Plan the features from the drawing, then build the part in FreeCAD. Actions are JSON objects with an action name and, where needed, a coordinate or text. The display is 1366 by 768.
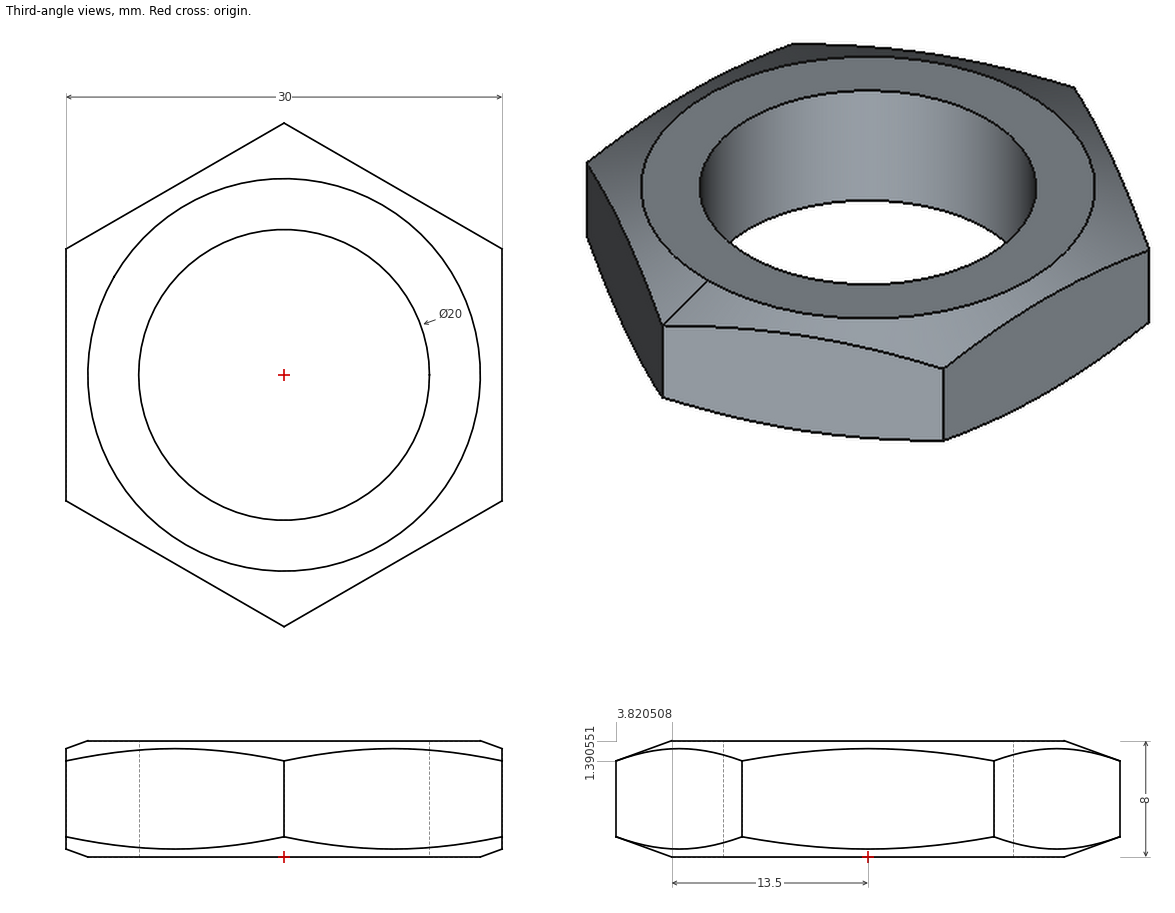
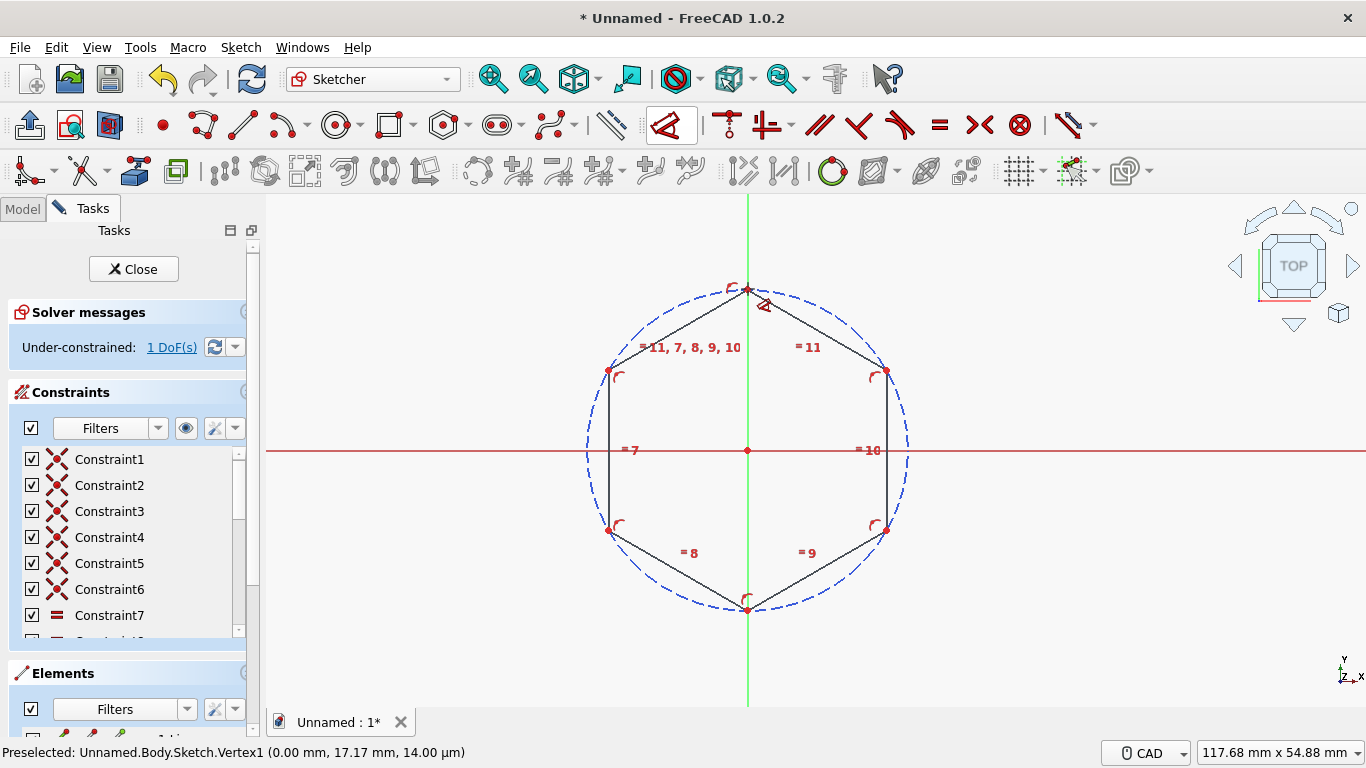
{"action": "left_click", "coordinate": [609, 370]}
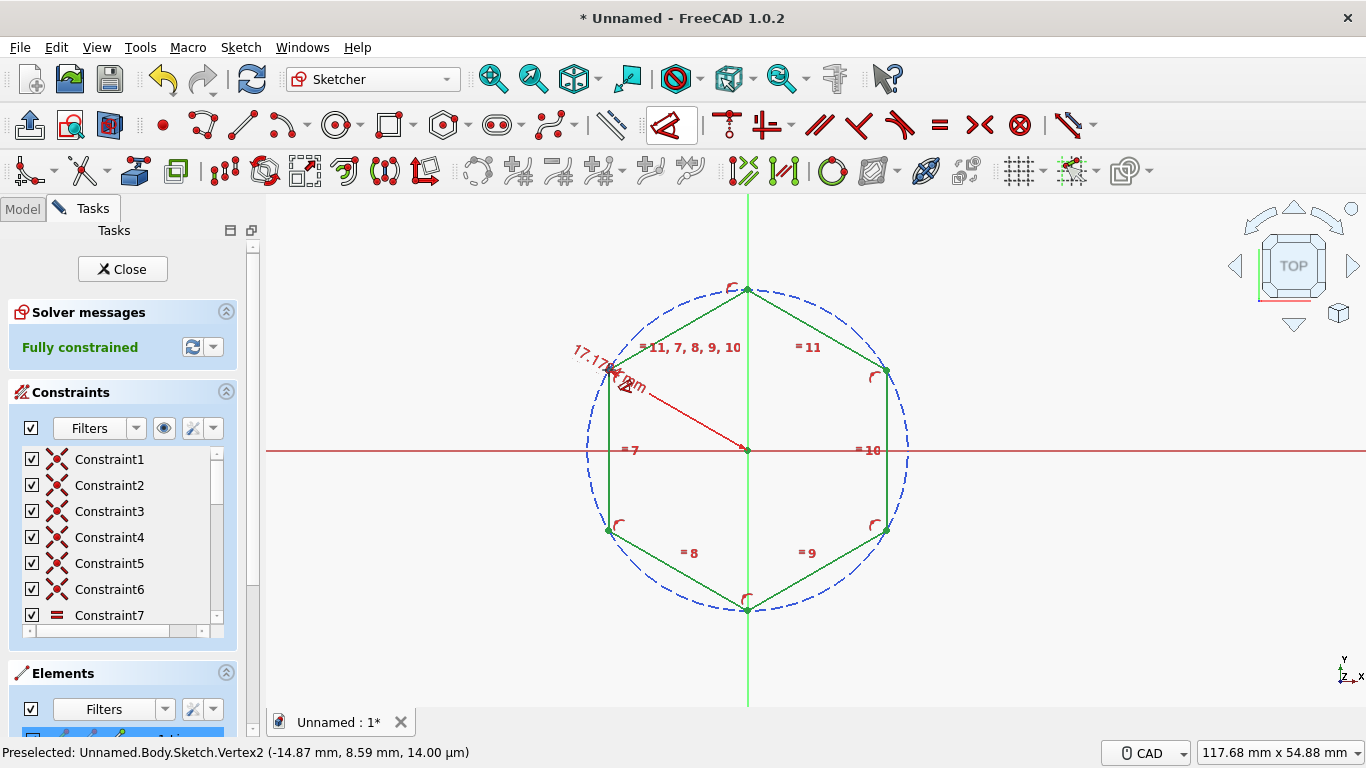
{"action": "left_click", "coordinate": [887, 531]}
{"action": "left_click", "coordinate": [684, 613]}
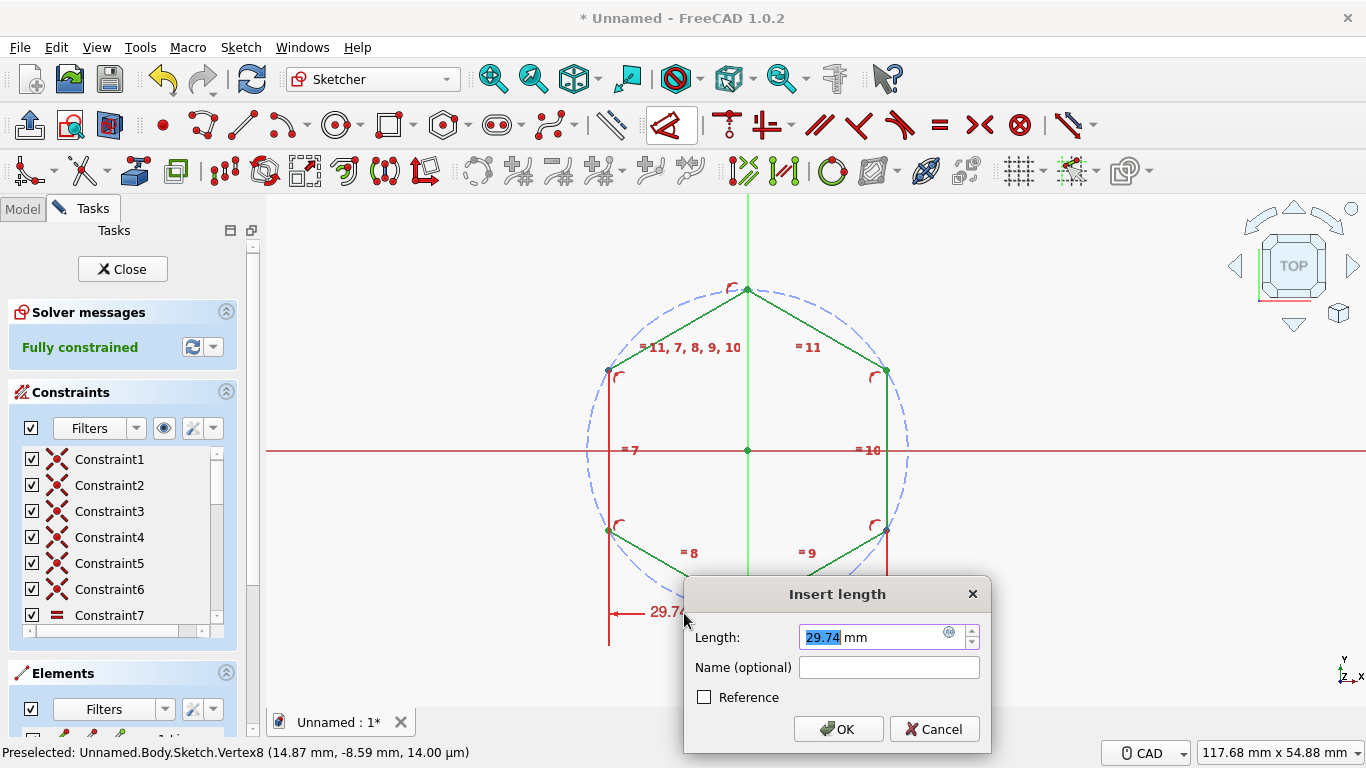
{"action": "type", "text": "30"}
{"action": "key", "text": "Return"}
{"action": "key", "text": "Escape"}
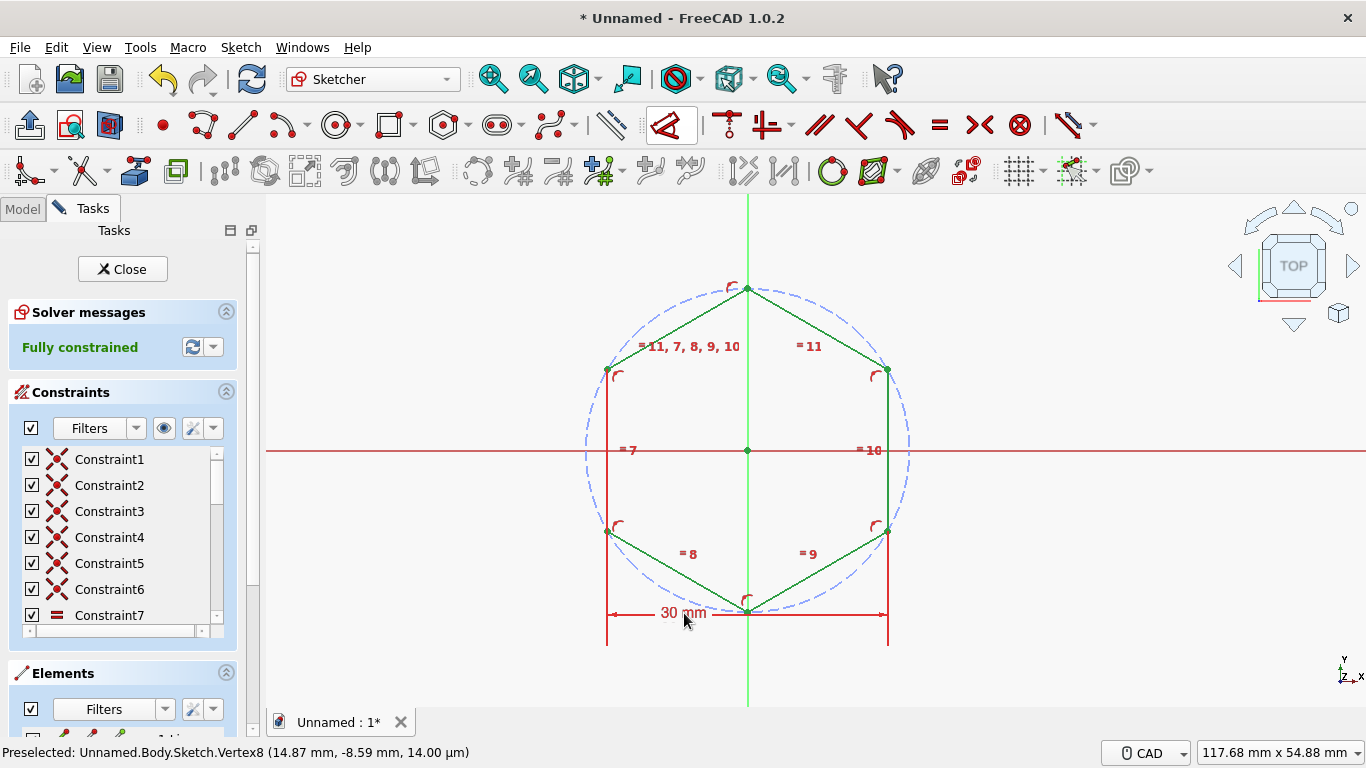
{"action": "left_click", "coordinate": [123, 269]}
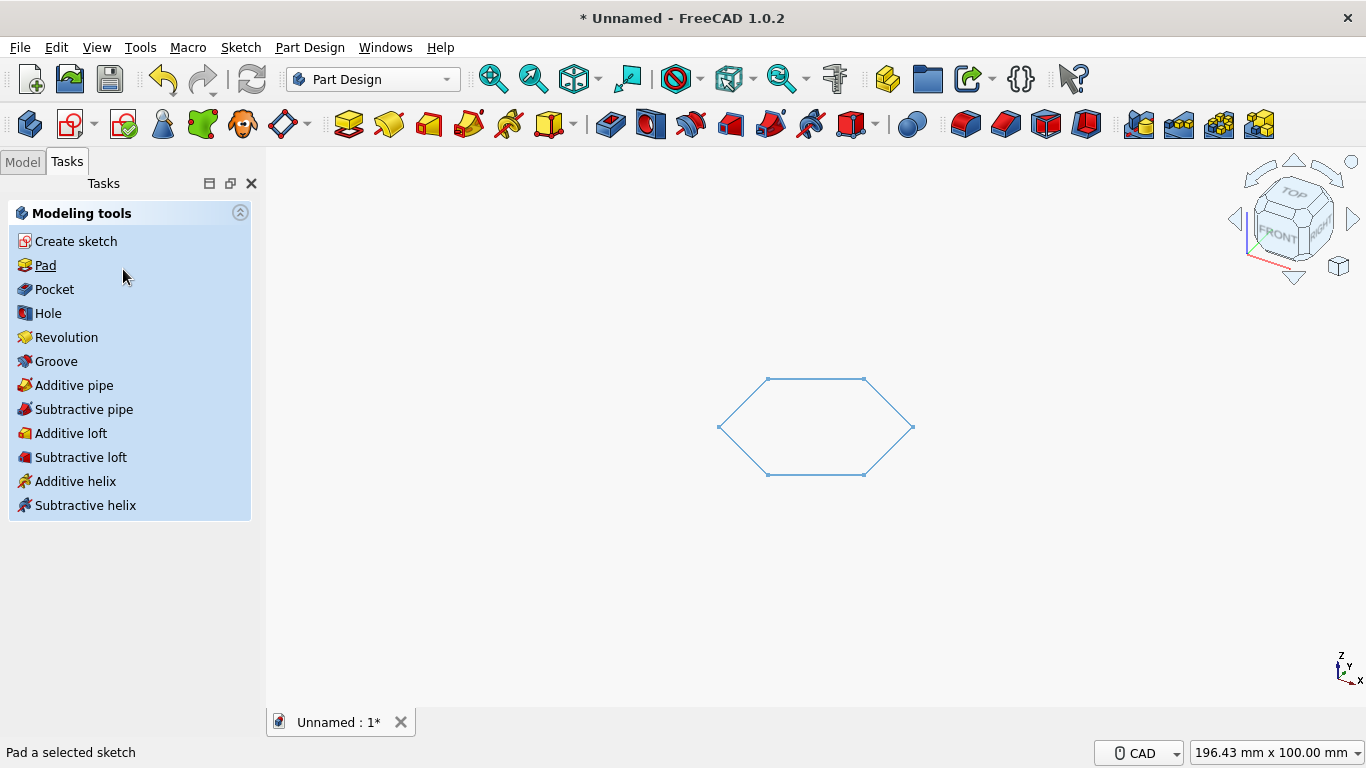
{"action": "left_click", "coordinate": [350, 124]}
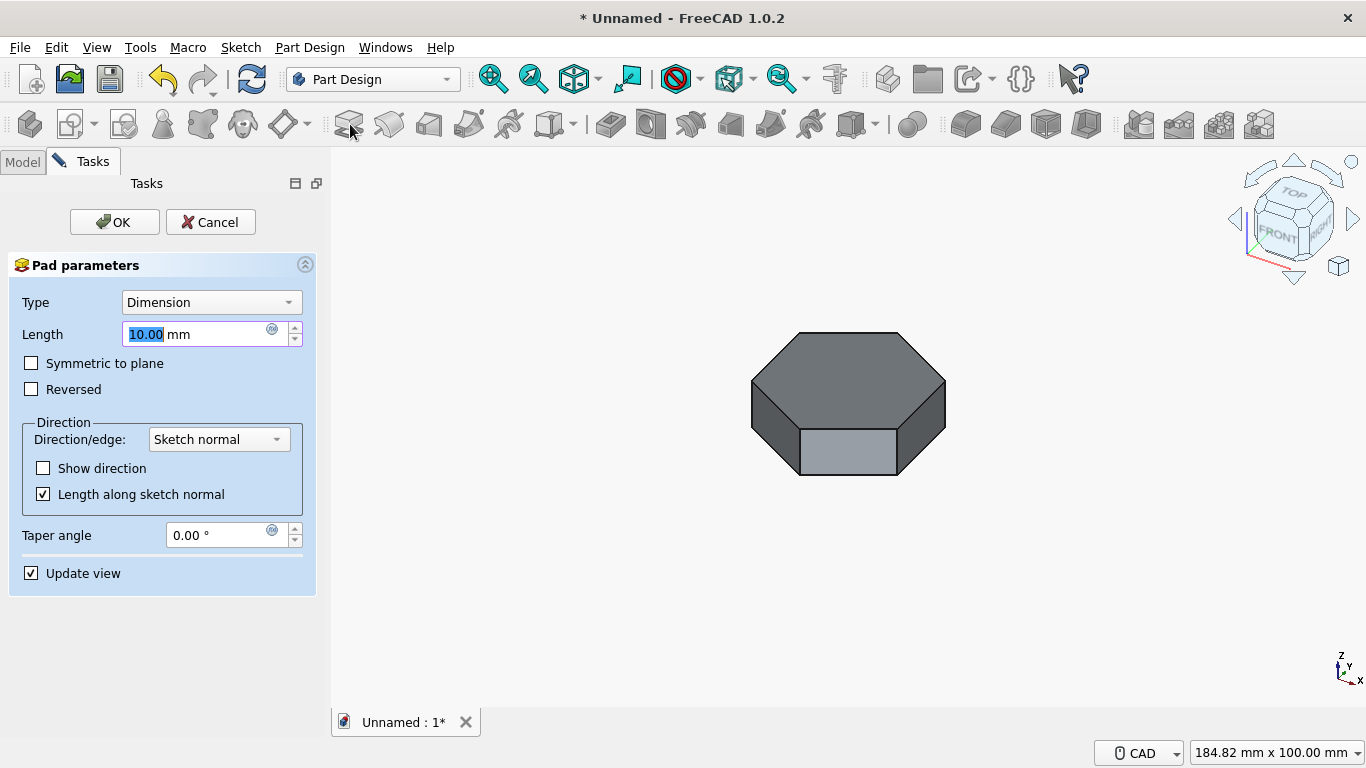
{"action": "type", "text": "8"}
{"action": "key", "text": "Tab"}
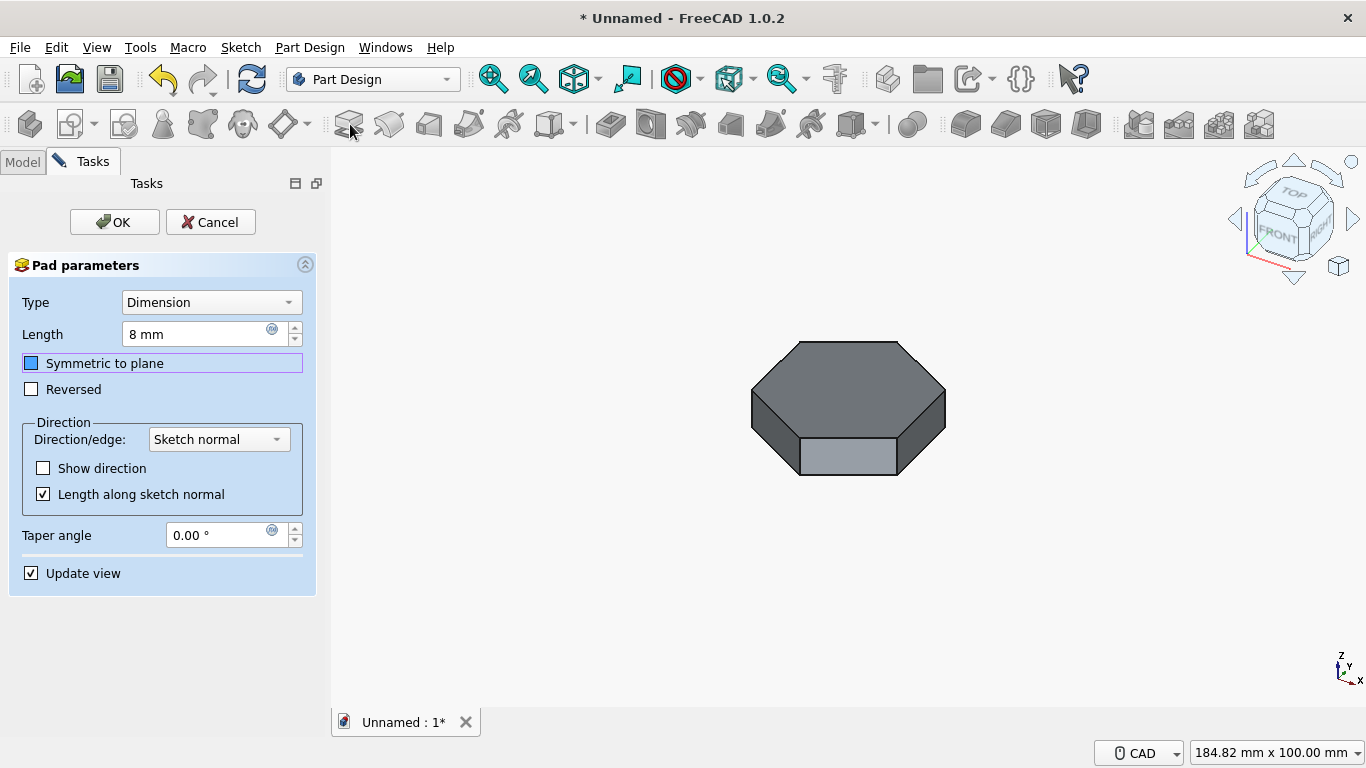
{"action": "left_click", "coordinate": [115, 222]}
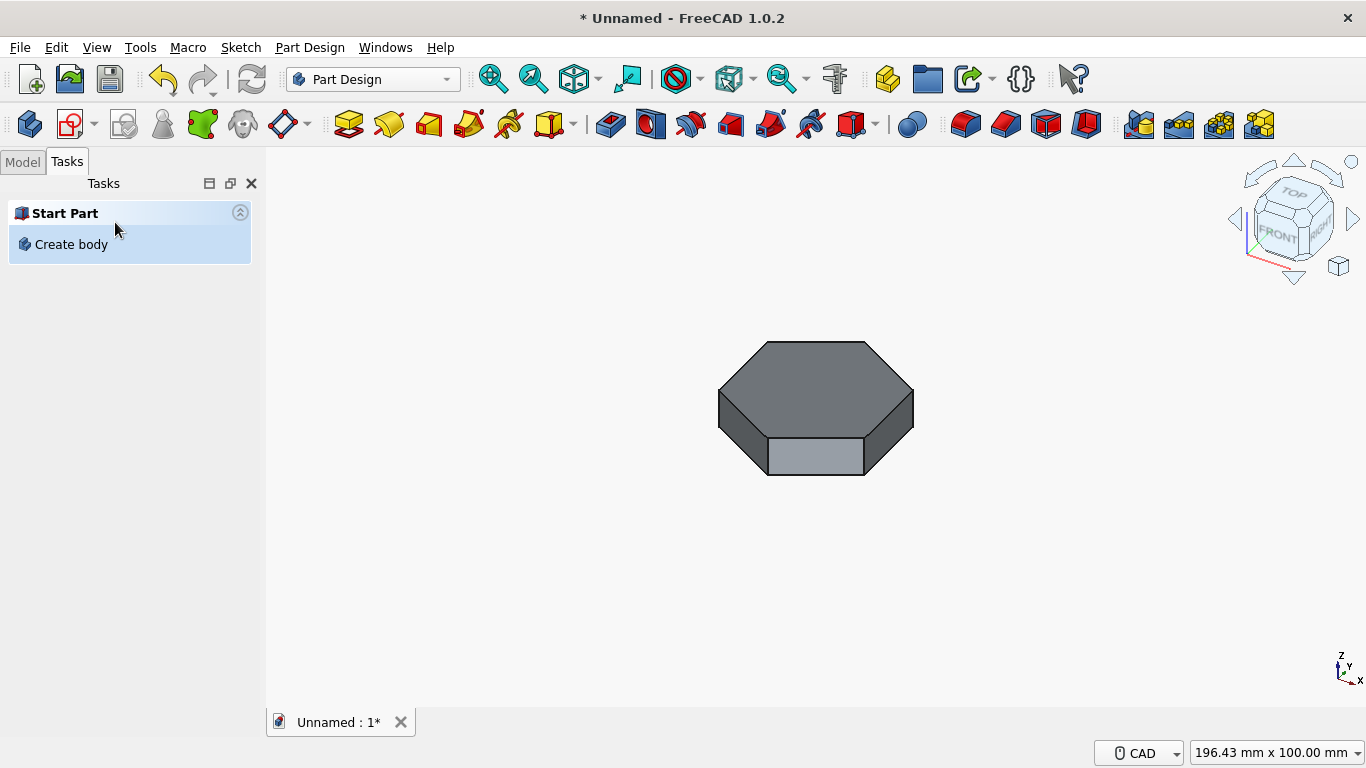
{"action": "left_click", "coordinate": [494, 80]}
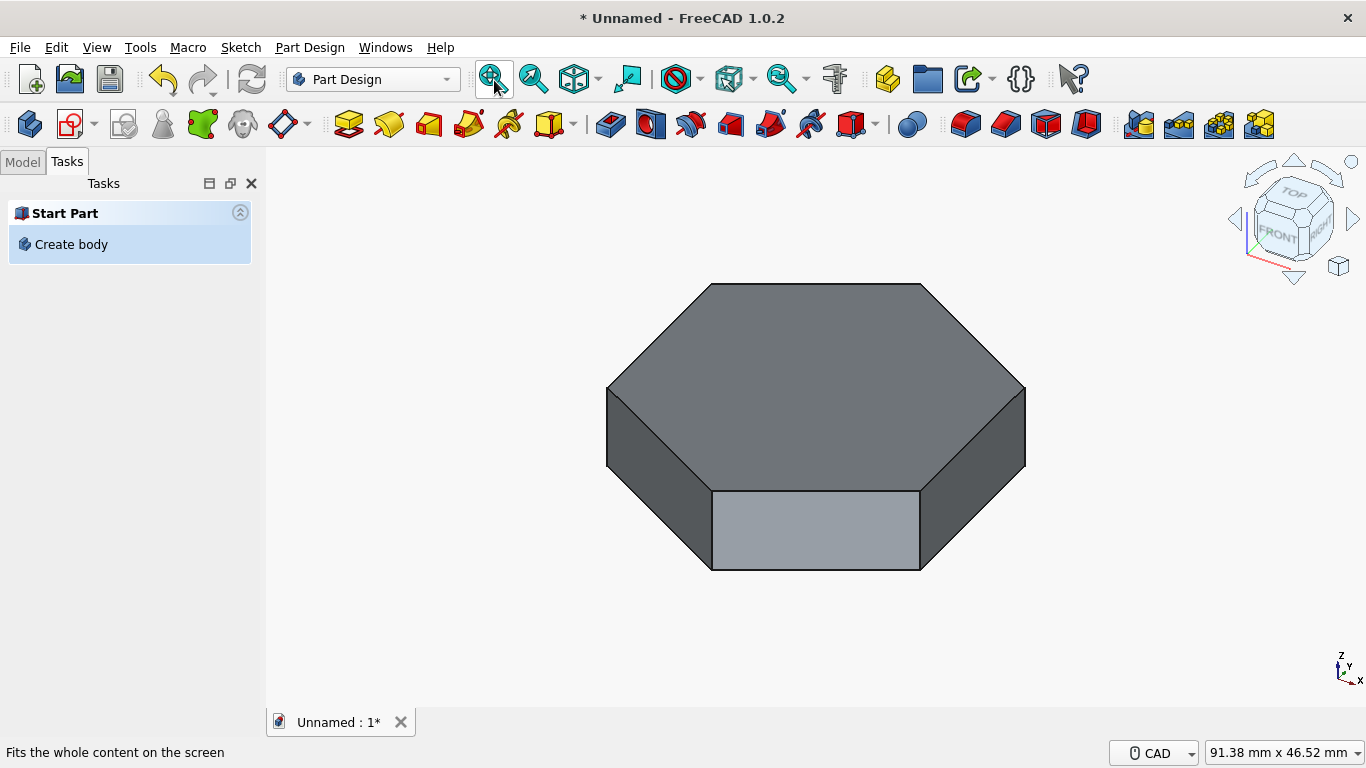
{"action": "left_click", "coordinate": [70, 124]}